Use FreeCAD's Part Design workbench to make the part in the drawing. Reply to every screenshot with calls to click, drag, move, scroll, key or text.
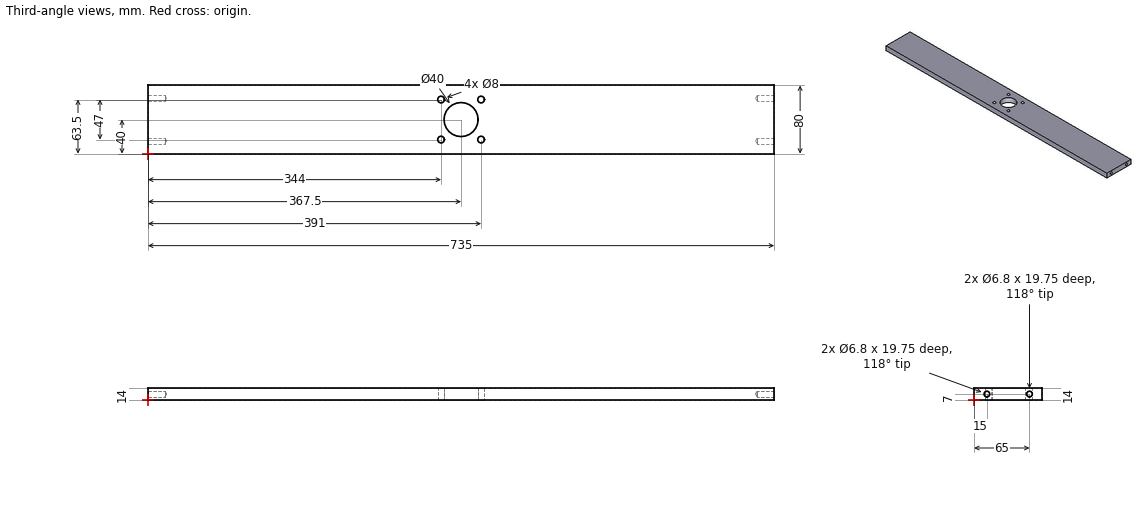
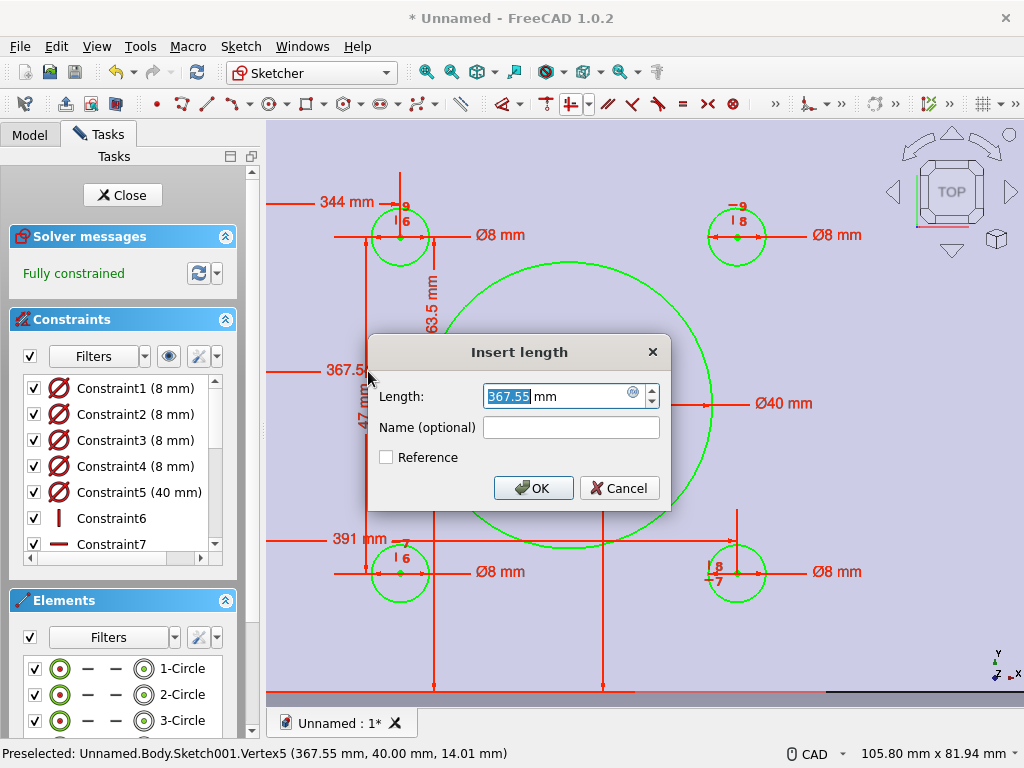
text(367.5)
key(Return)
key(Escape)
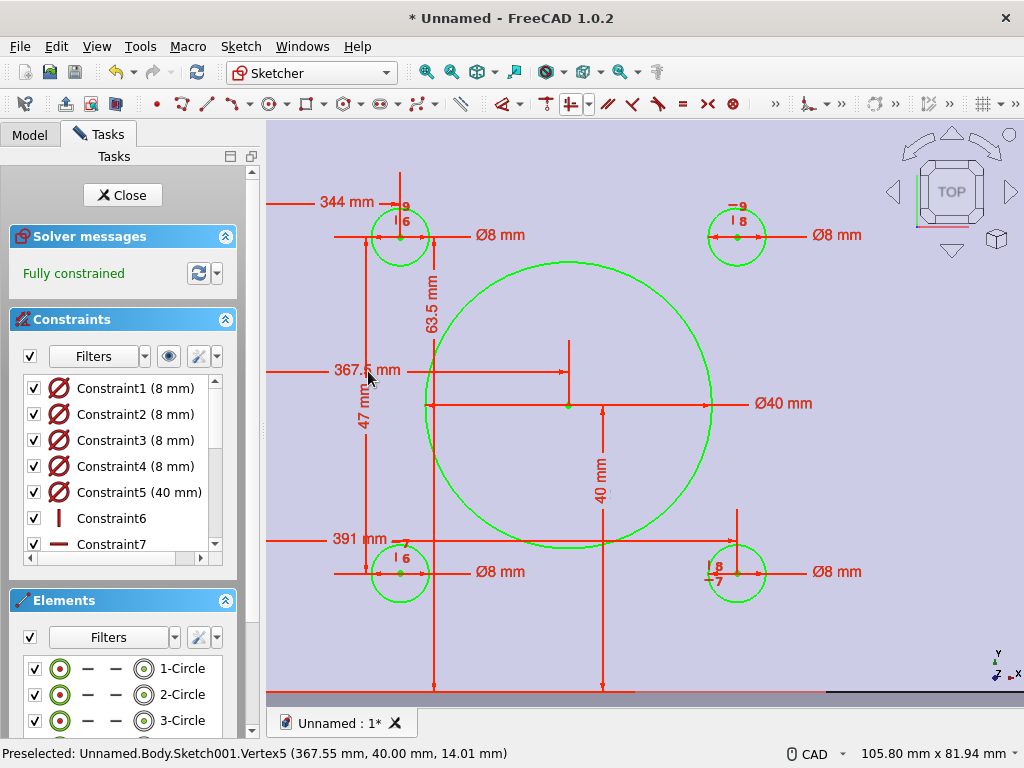
click(123, 195)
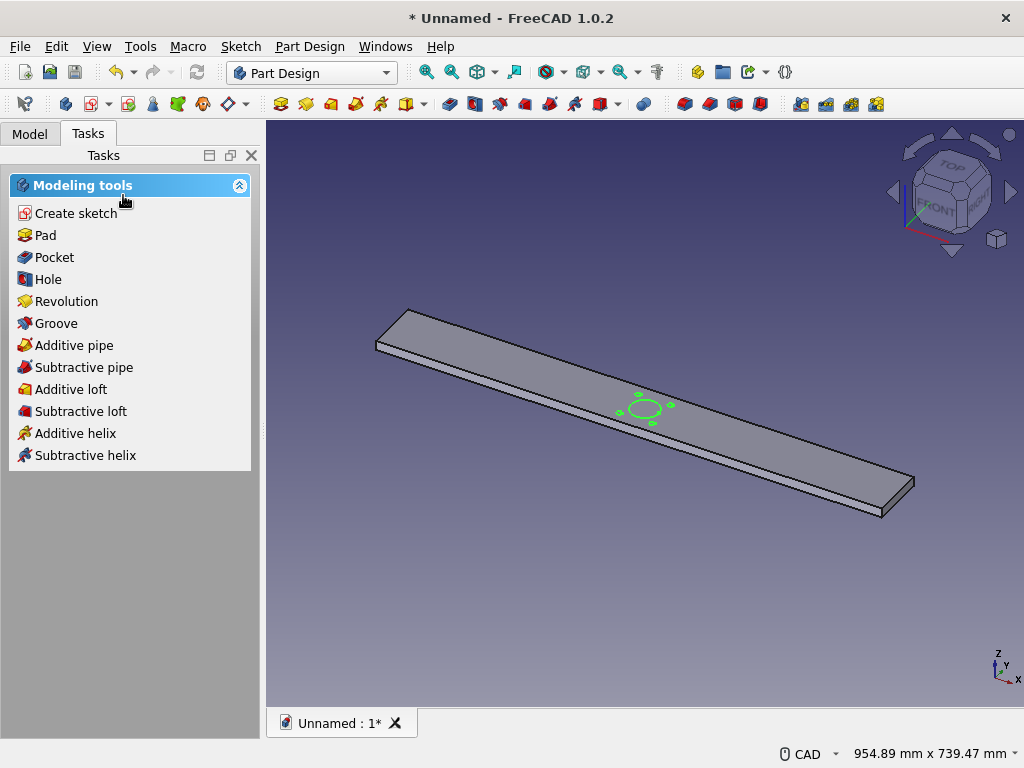
click(450, 104)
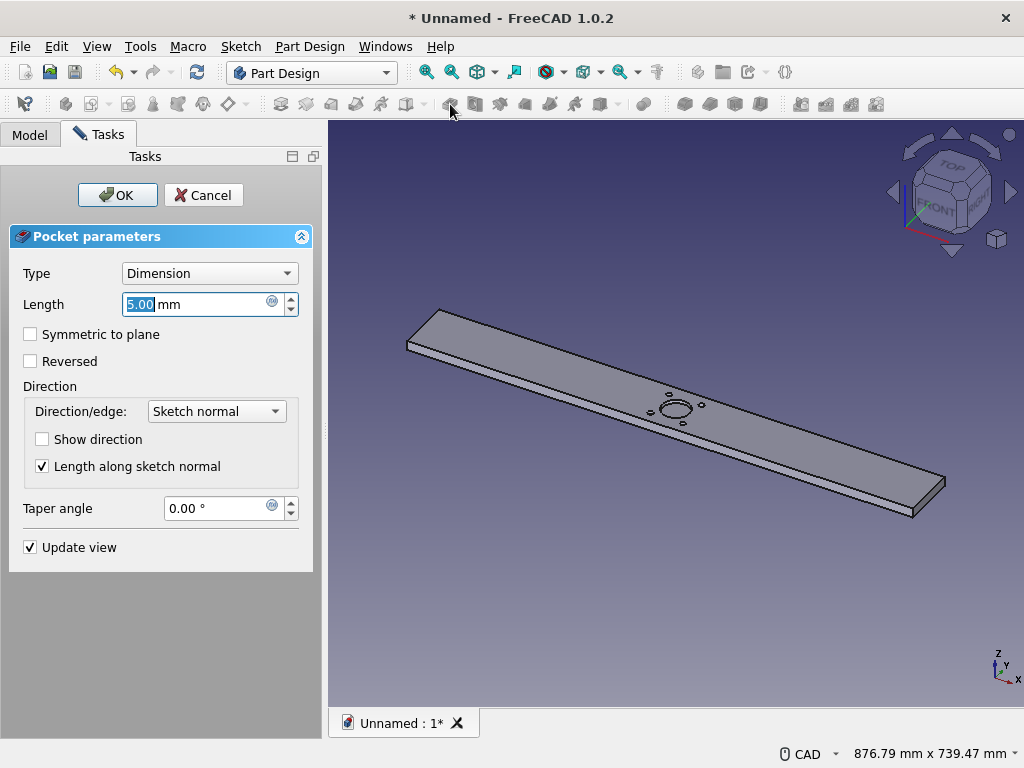
text(14)
key(Tab)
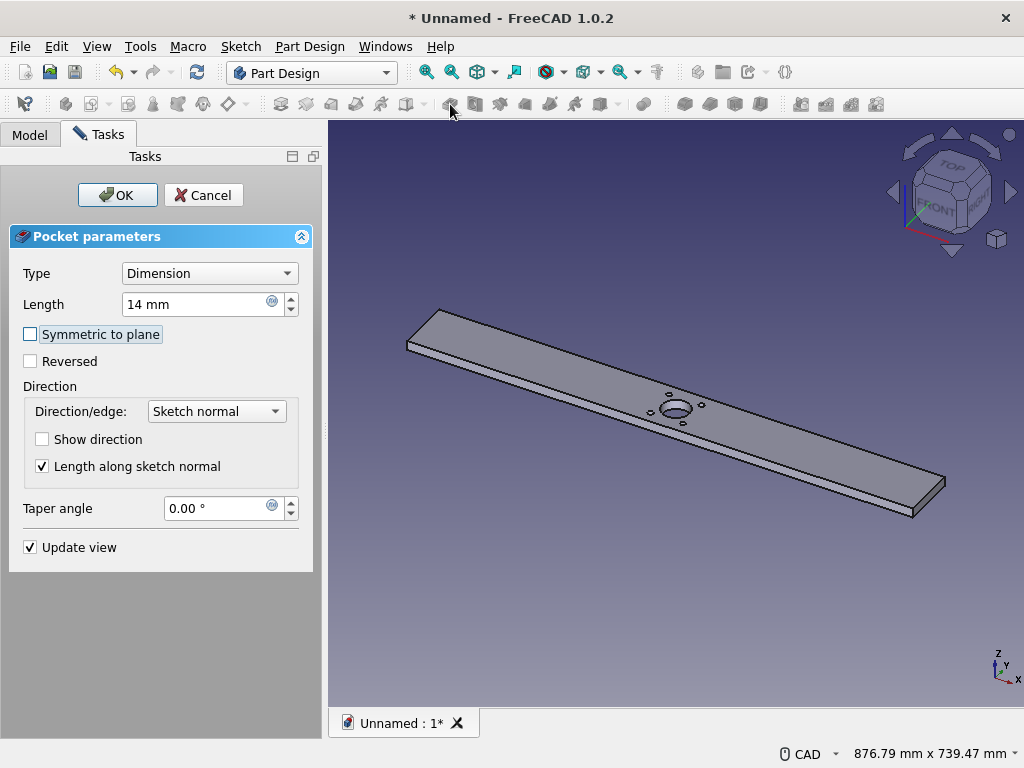
click(118, 195)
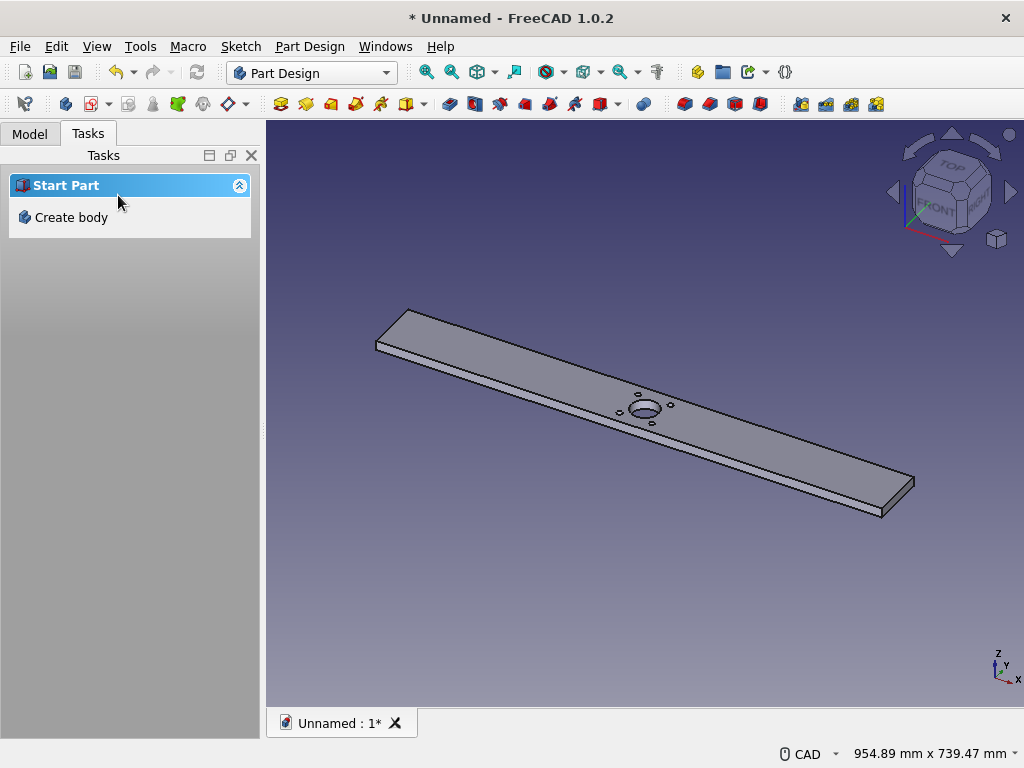
key(6)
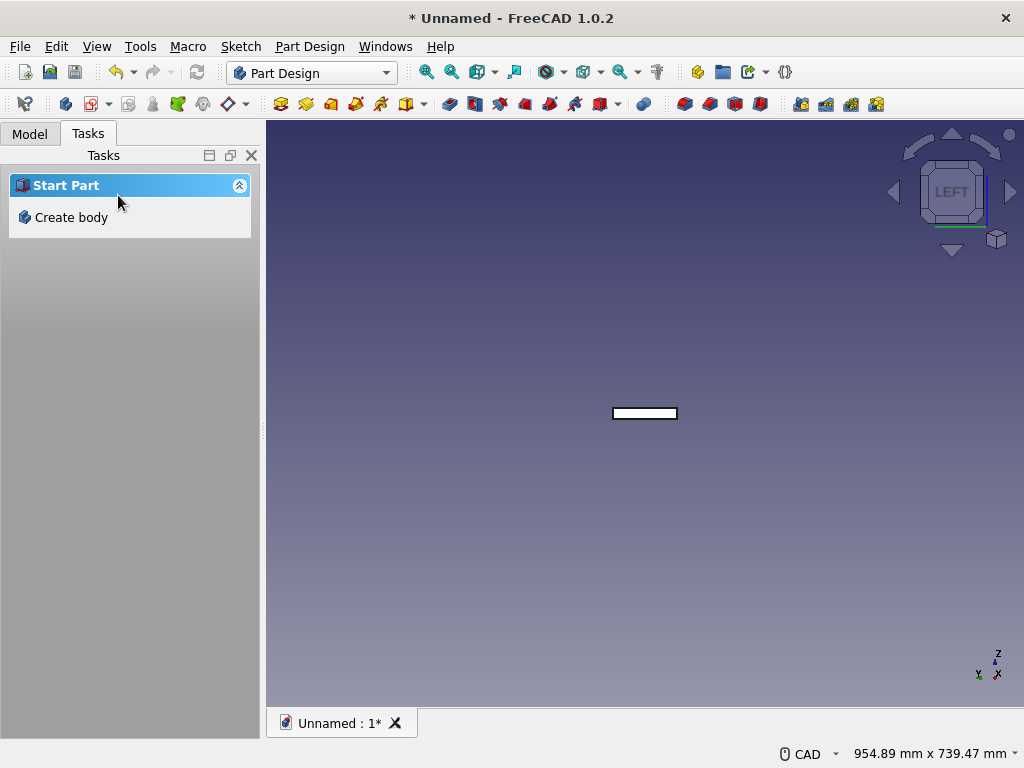
click(427, 72)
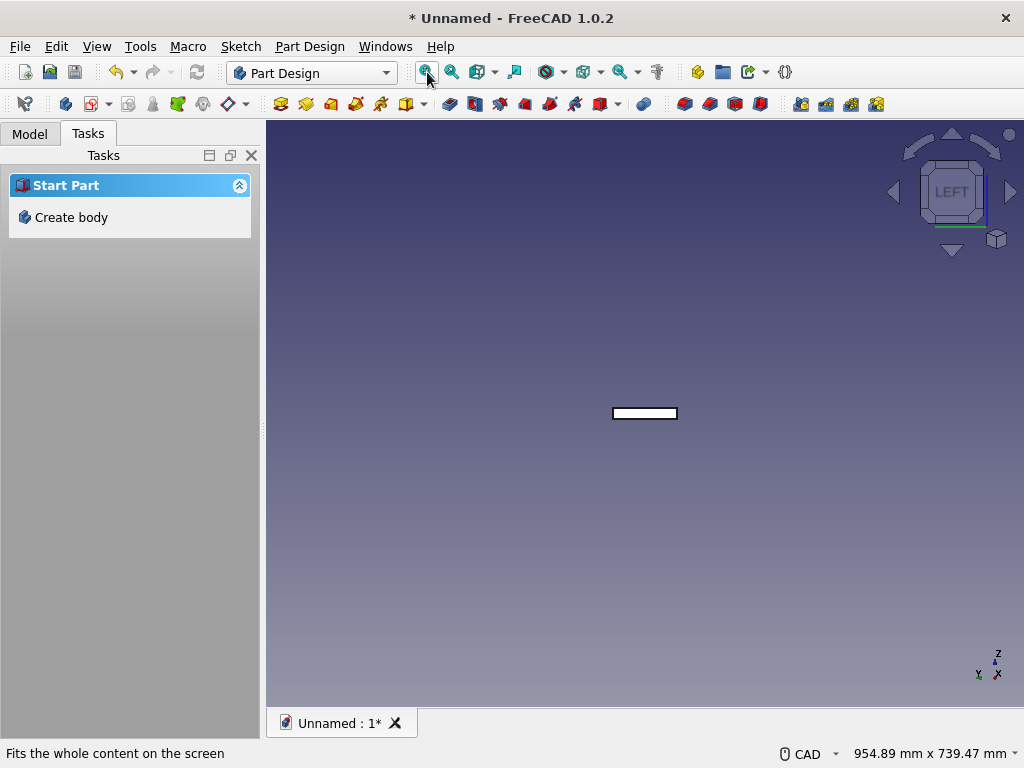
scroll(627, 412, up, 4)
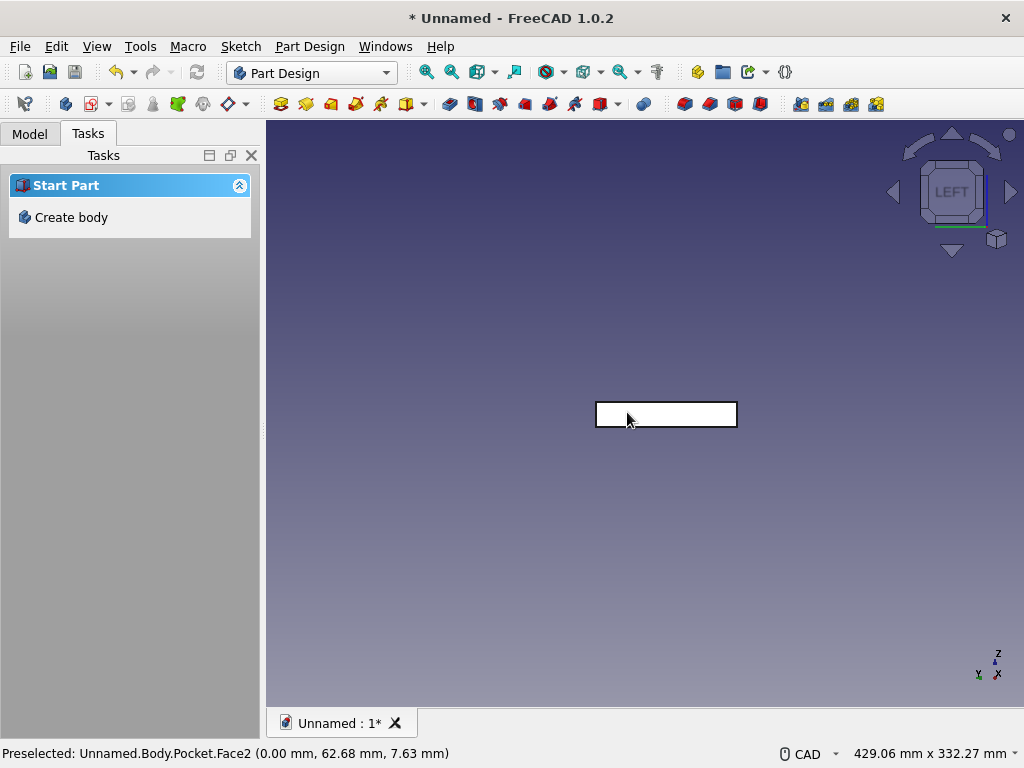
click(626, 414)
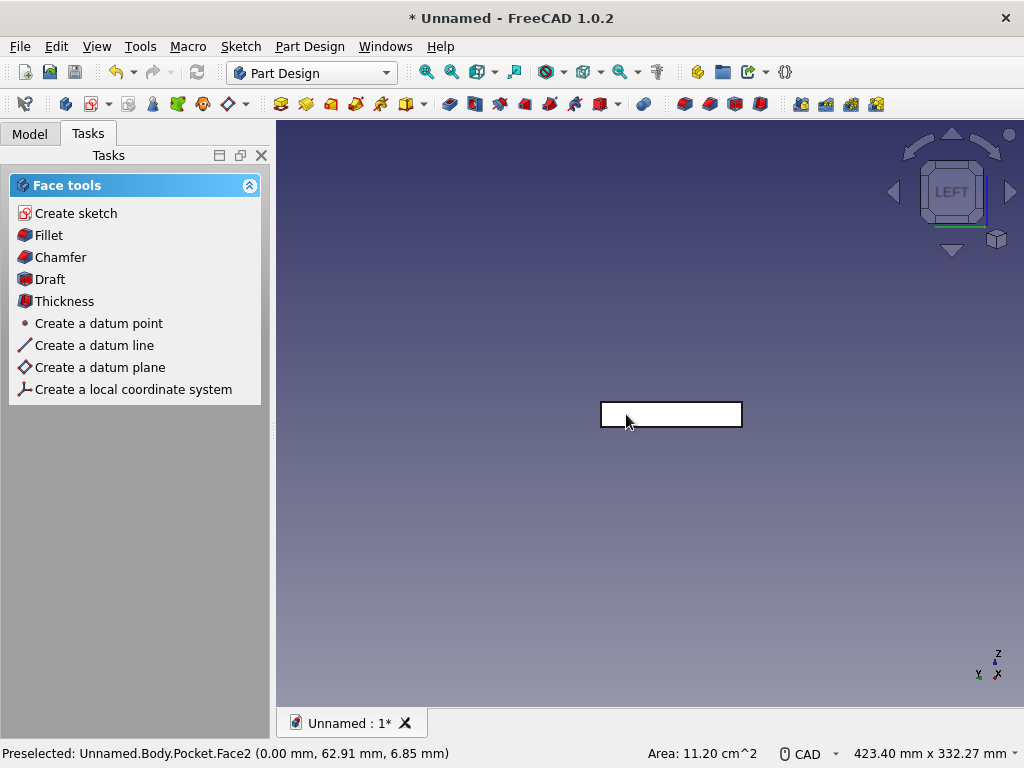
click(90, 104)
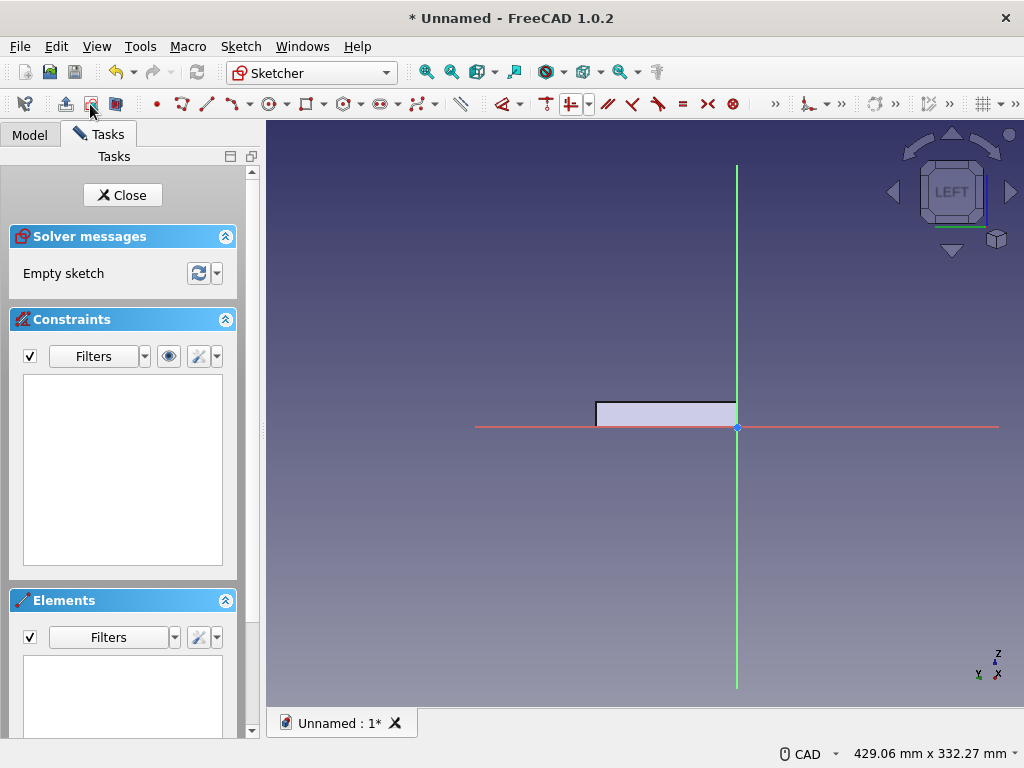
scroll(720, 420, up, 6)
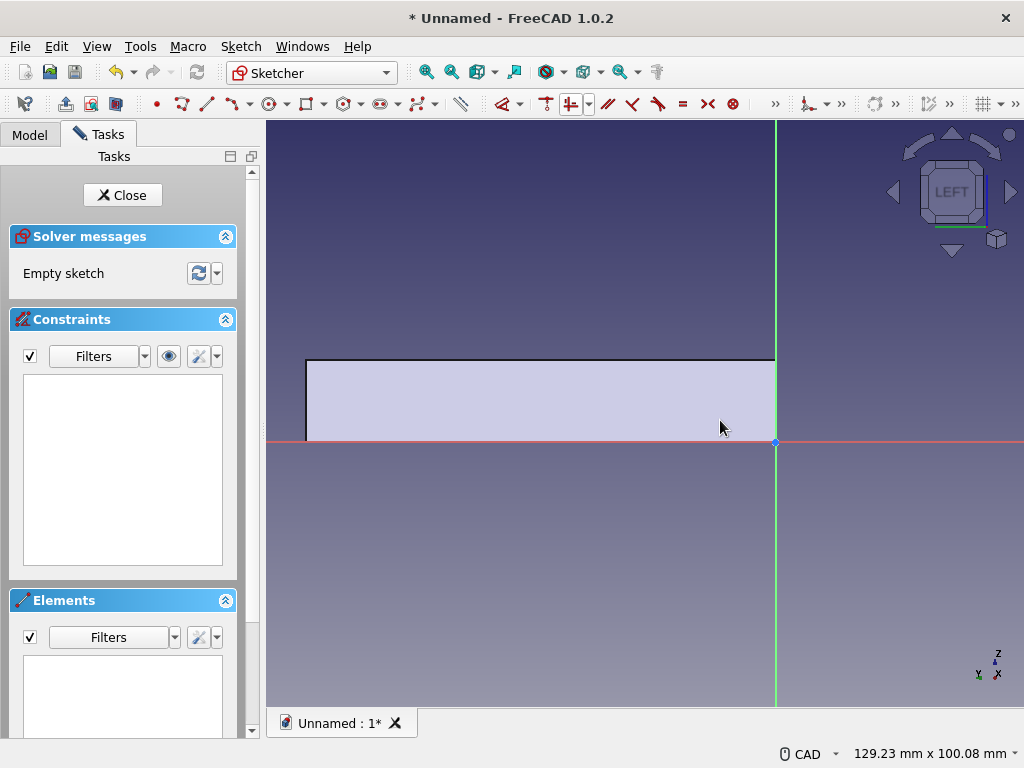
key(g)
key(c)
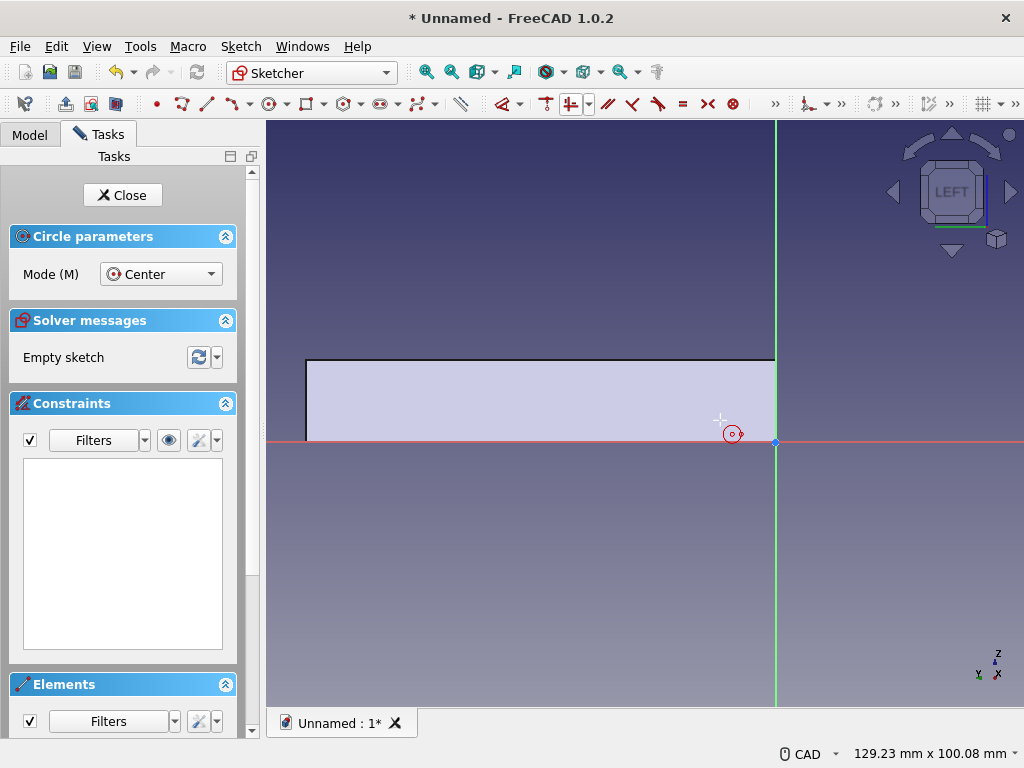
click(394, 401)
move(408, 387)